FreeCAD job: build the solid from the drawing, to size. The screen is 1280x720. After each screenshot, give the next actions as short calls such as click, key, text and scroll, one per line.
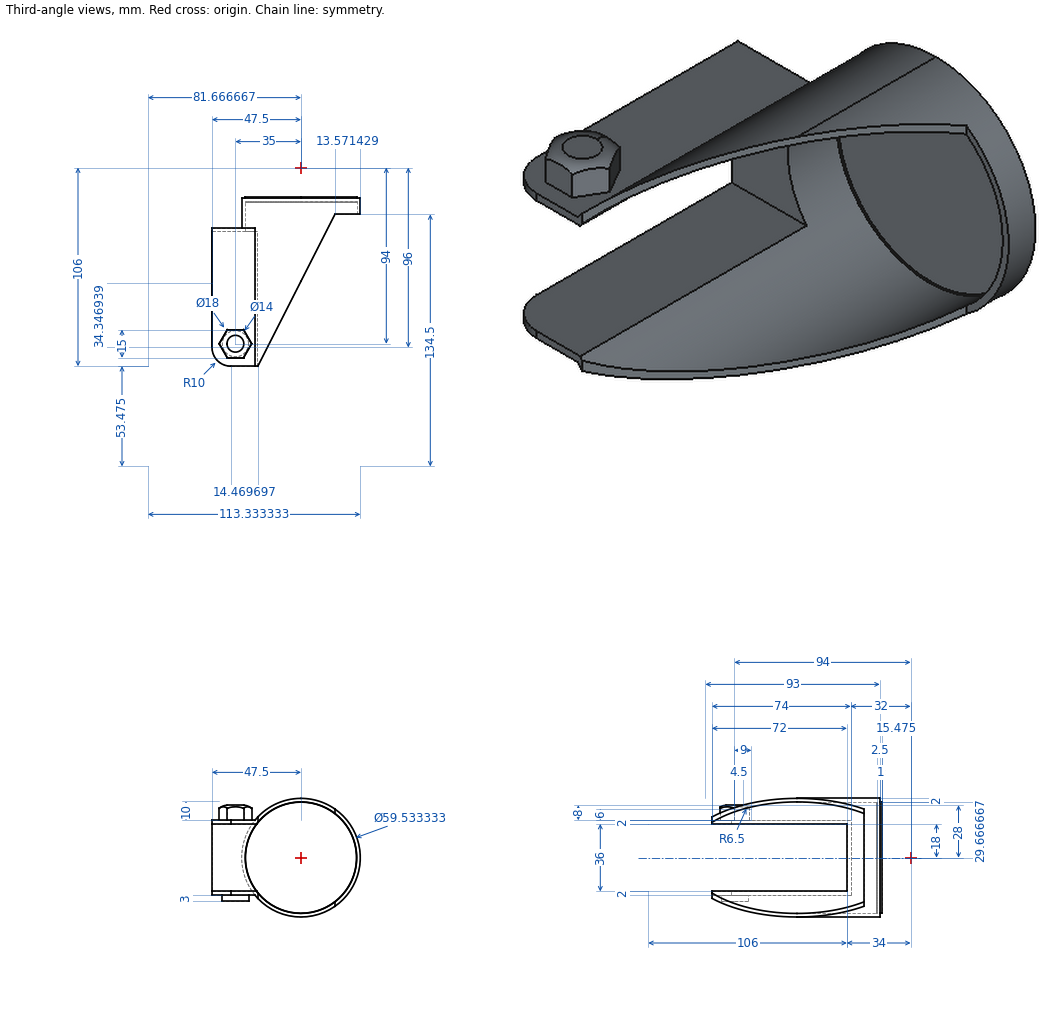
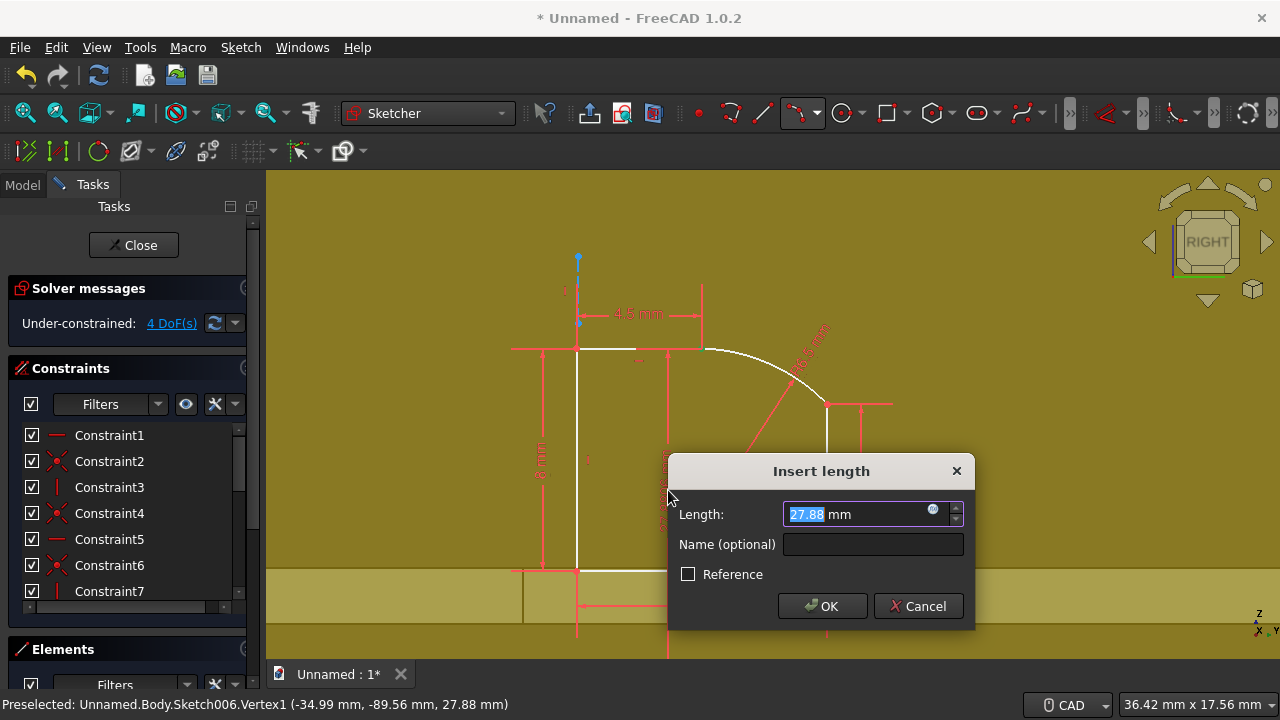
text(28)
key(Return)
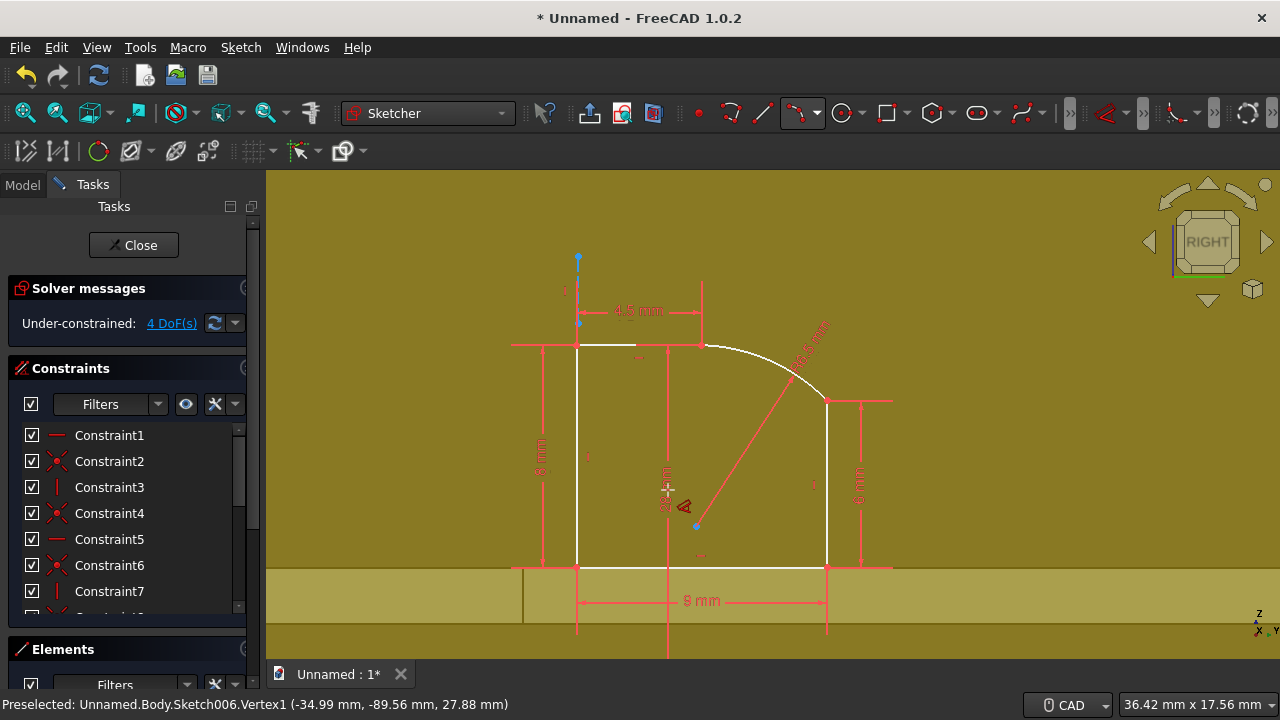
click(577, 345)
click(846, 311)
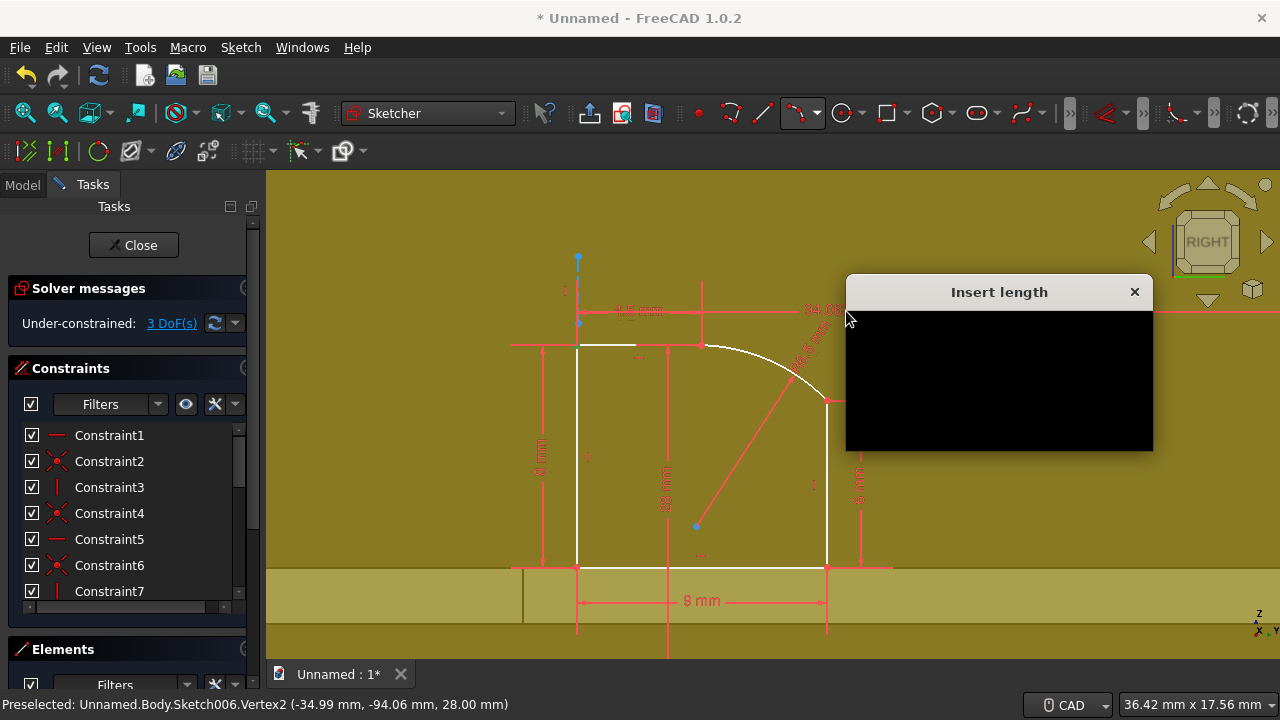
text(94)
key(Return)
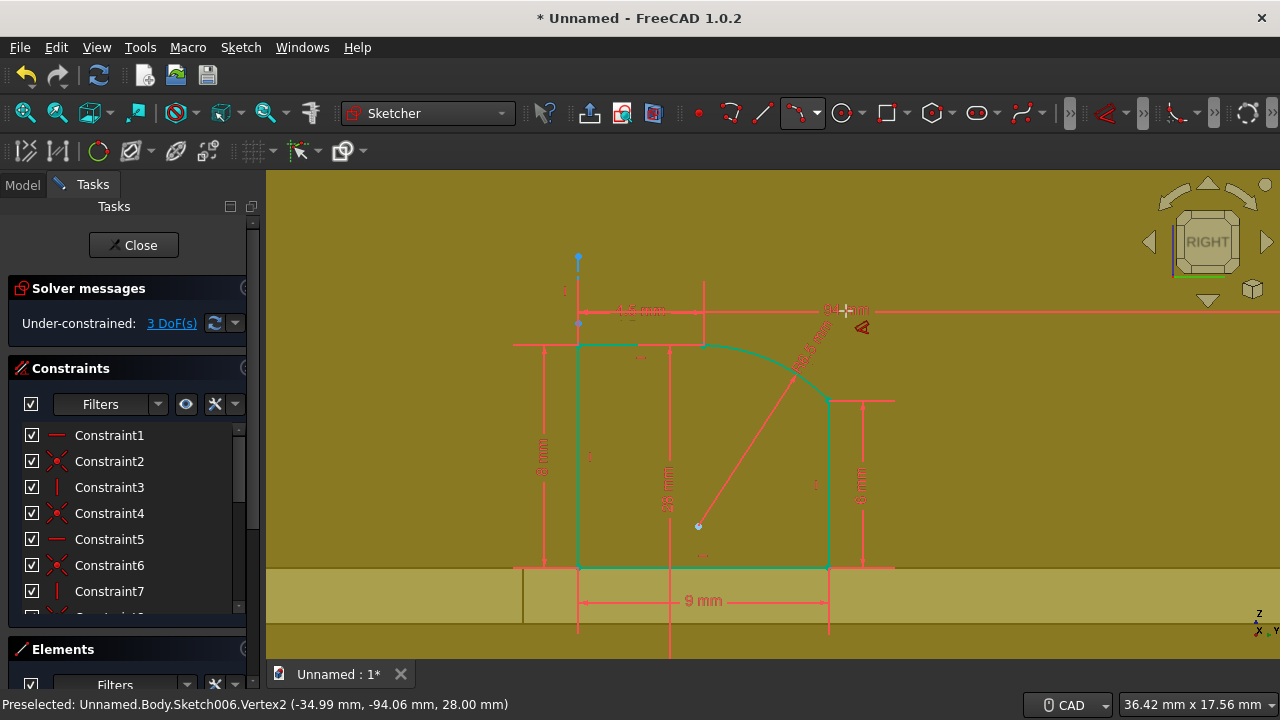
click(578, 324)
click(847, 290)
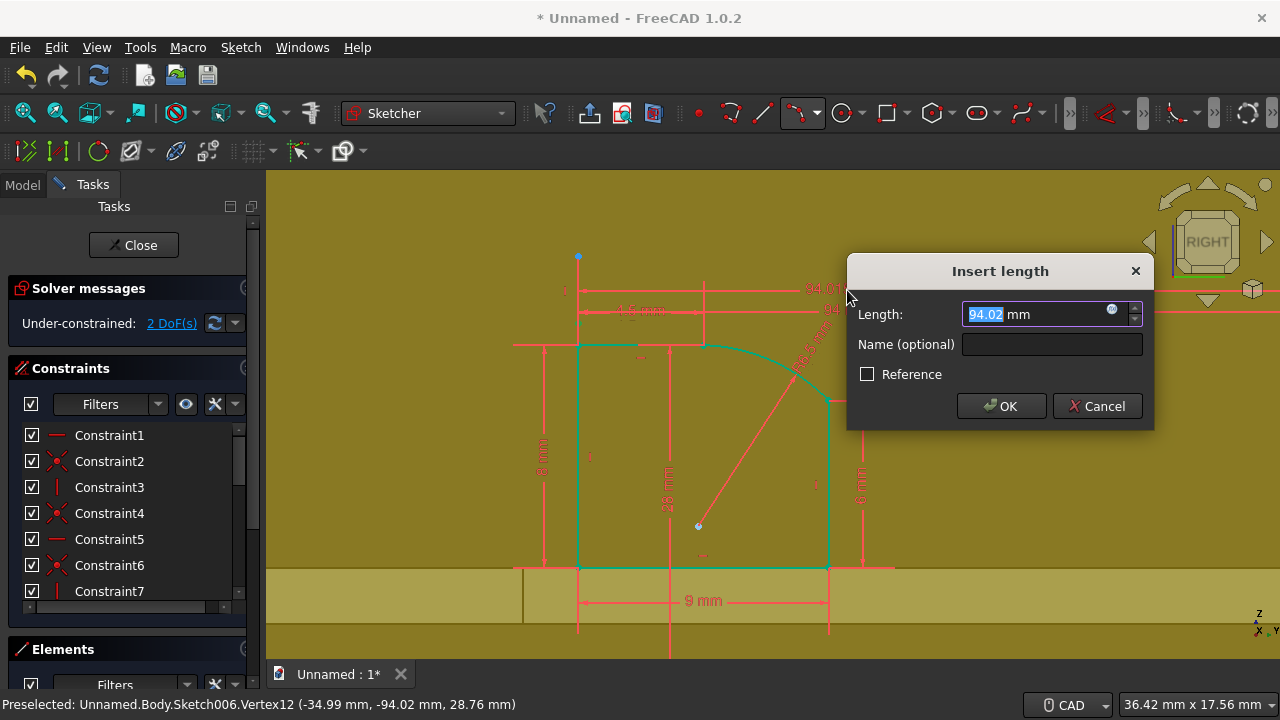
text(94)
key(Return)
key(Escape)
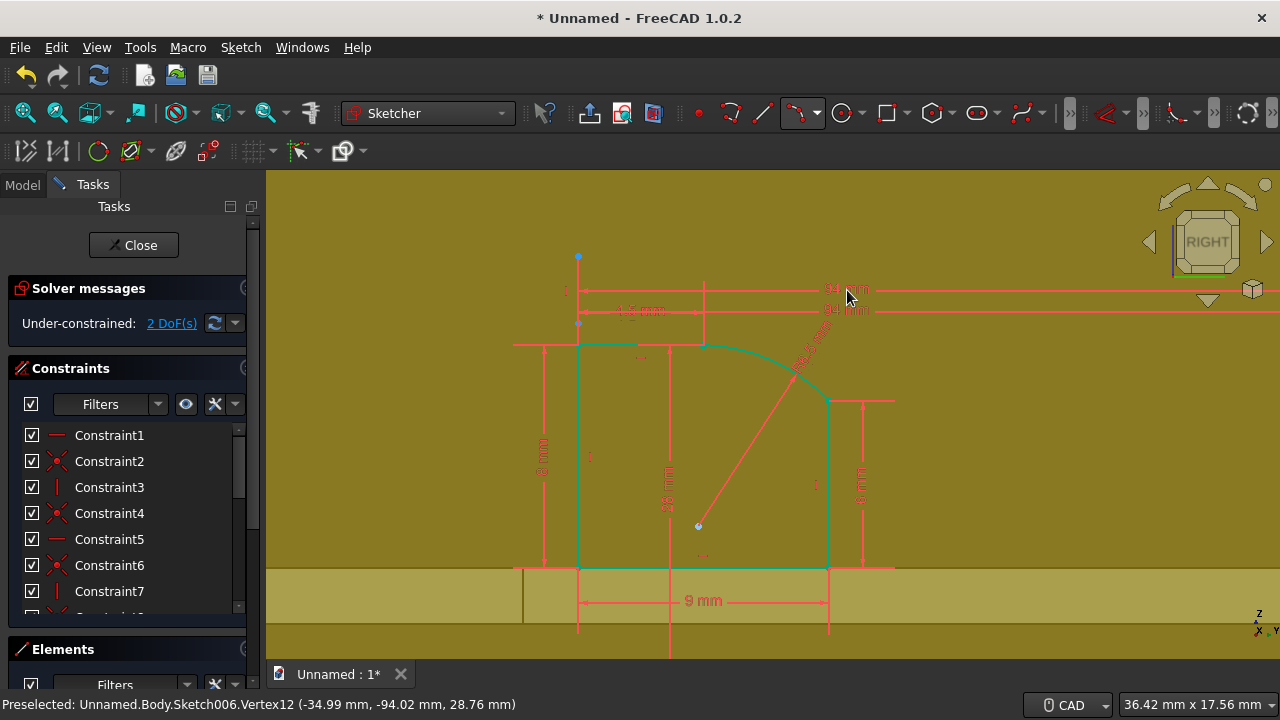
click(134, 245)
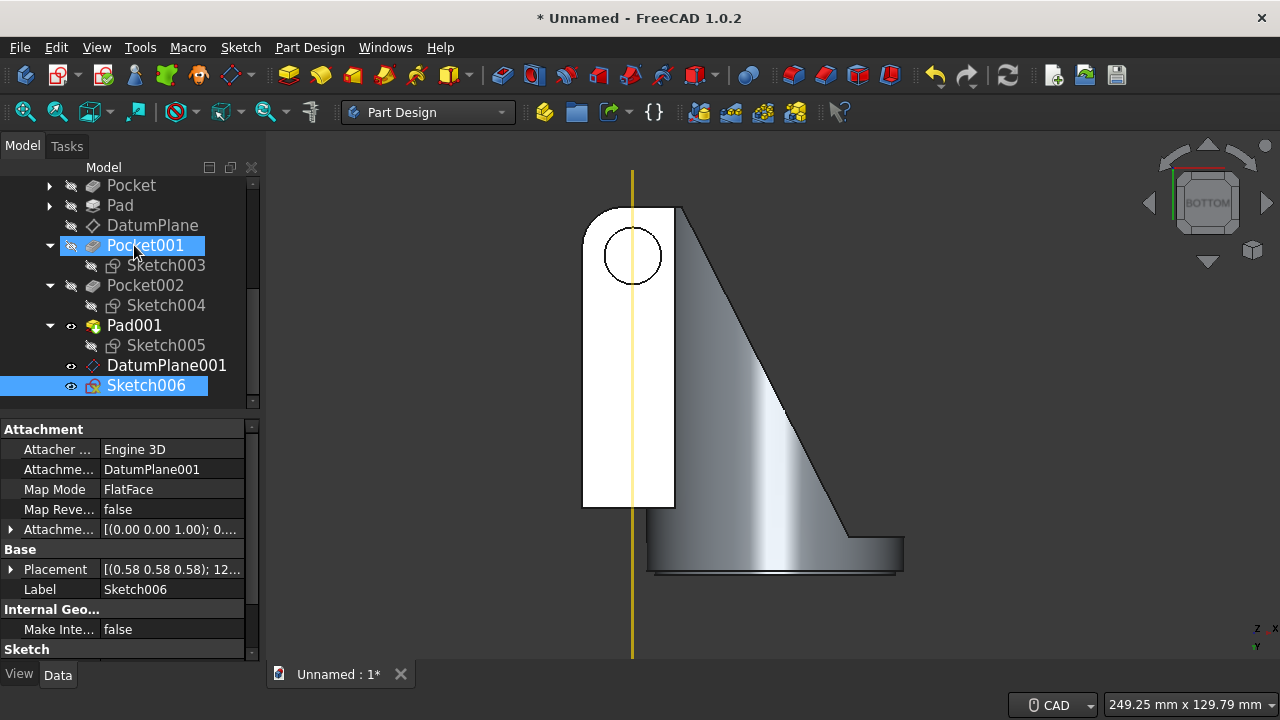
click(322, 76)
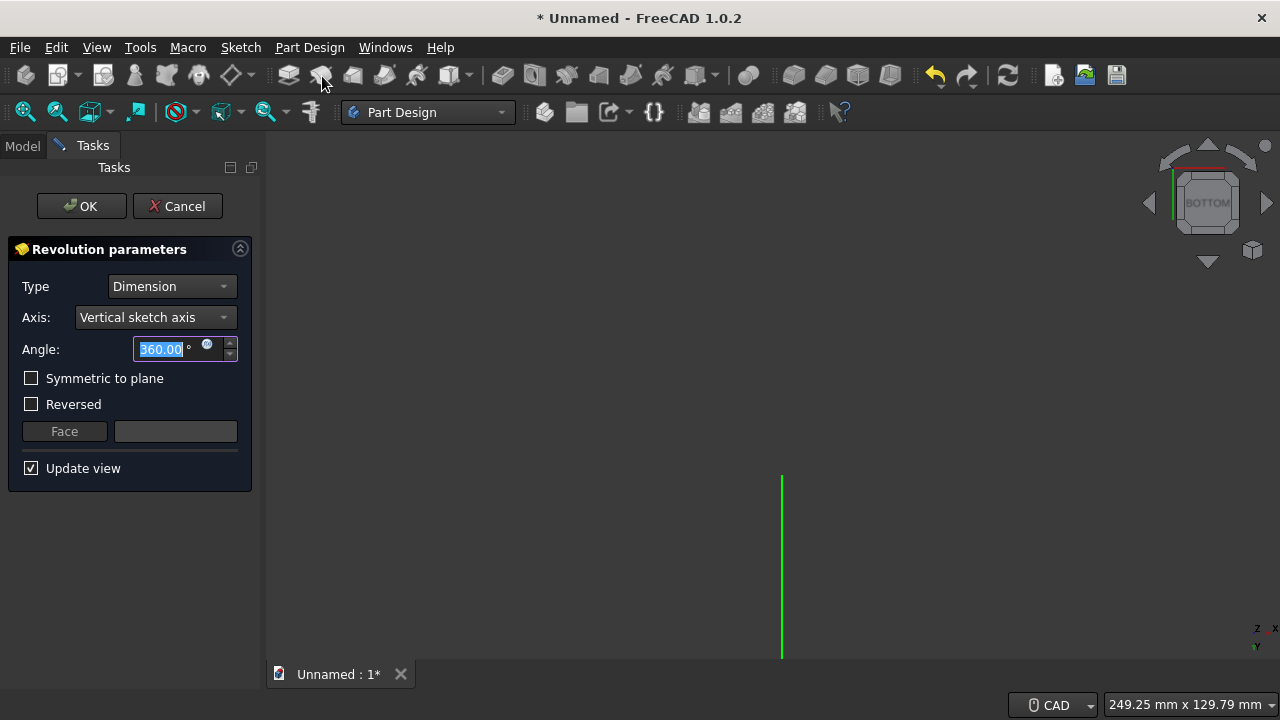
click(156, 318)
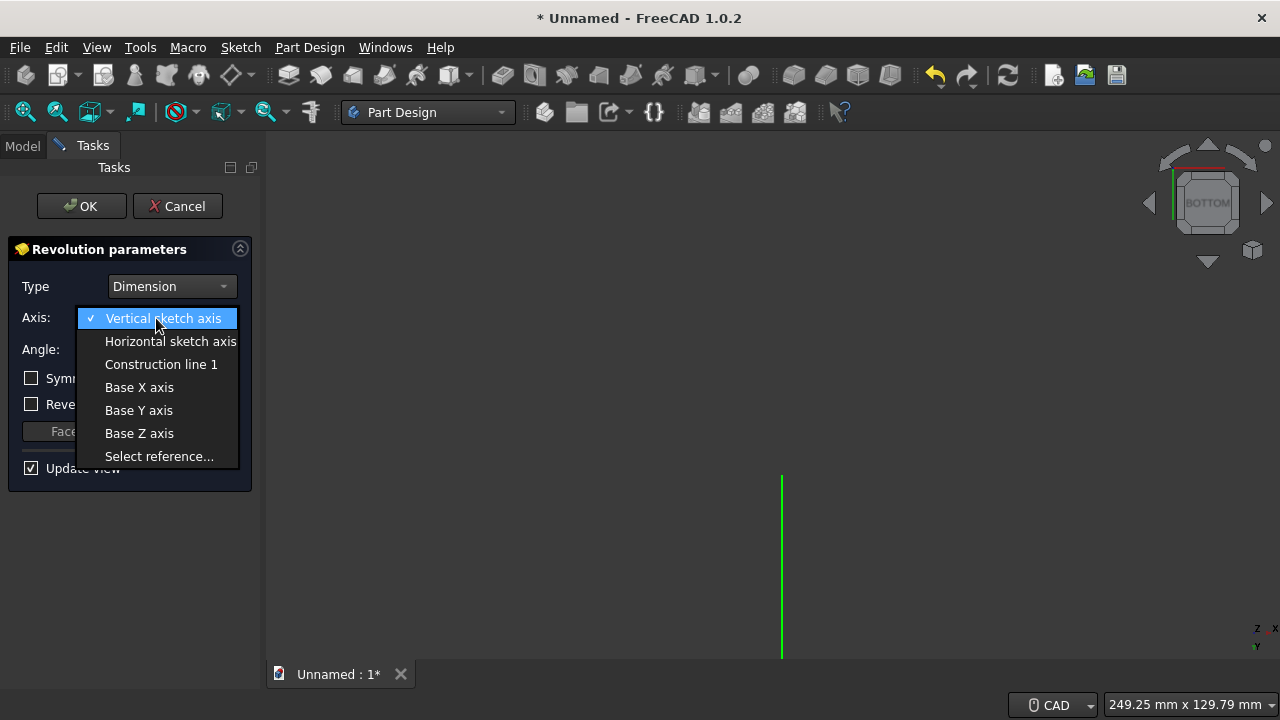
click(156, 364)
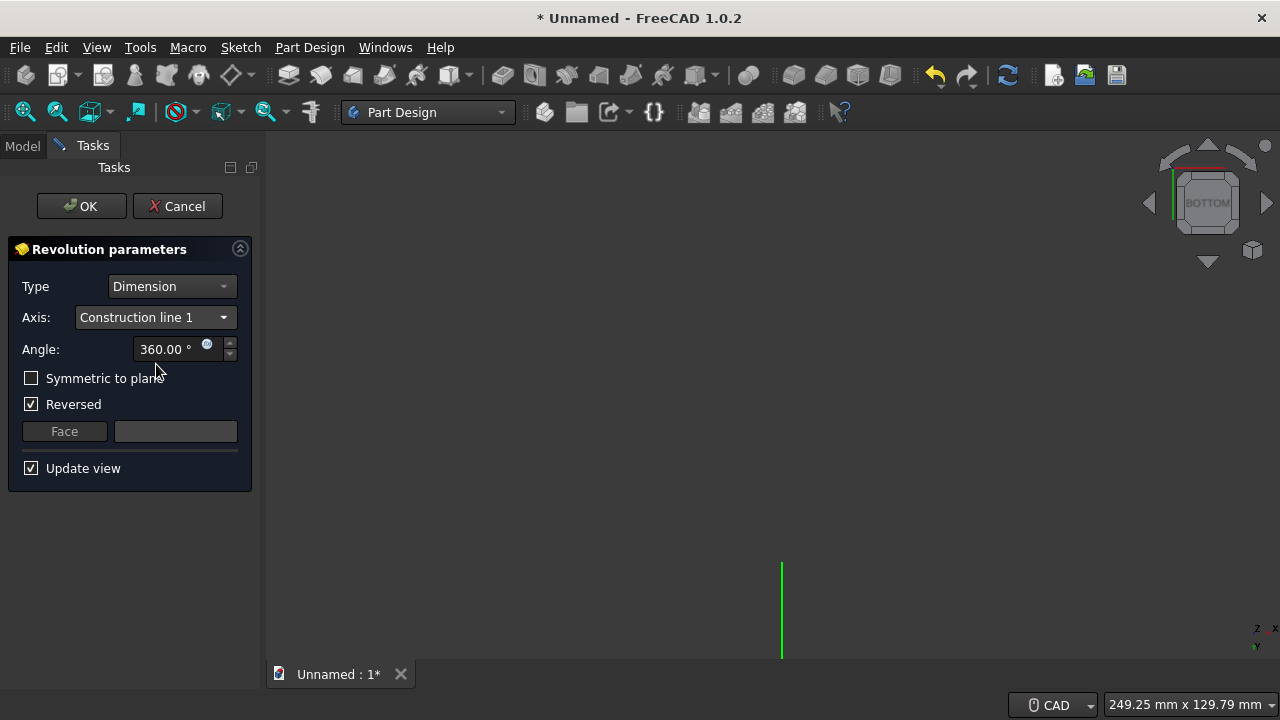
click(82, 206)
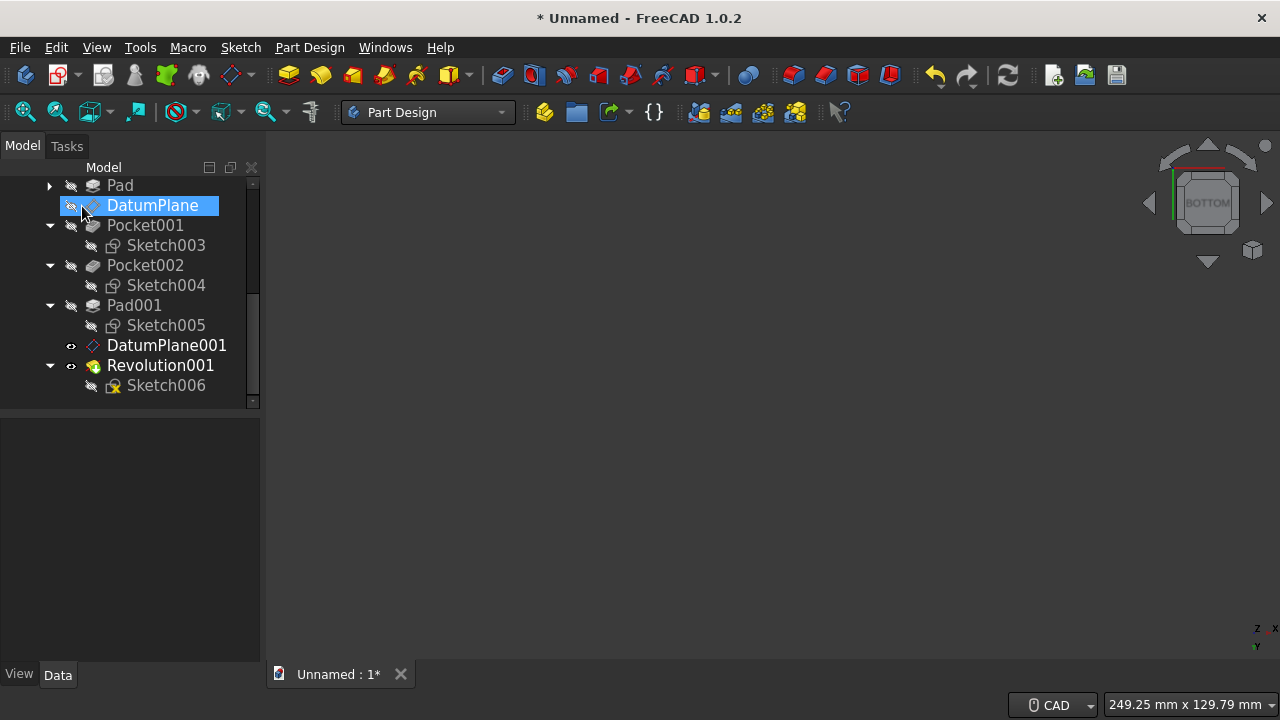
click(116, 346)
key(space)